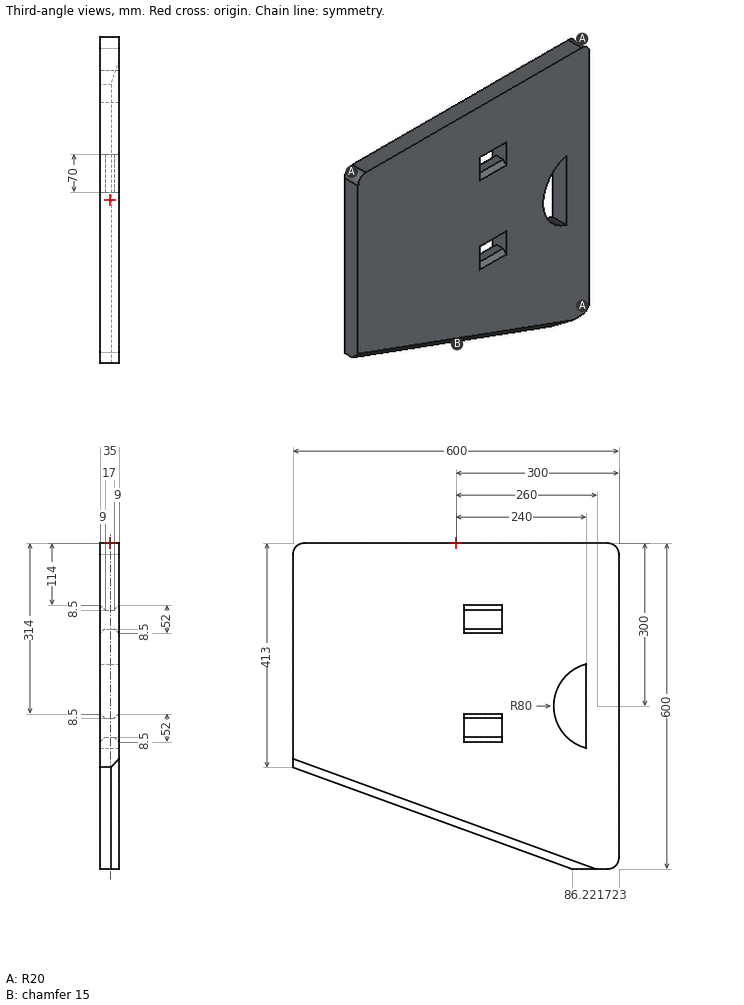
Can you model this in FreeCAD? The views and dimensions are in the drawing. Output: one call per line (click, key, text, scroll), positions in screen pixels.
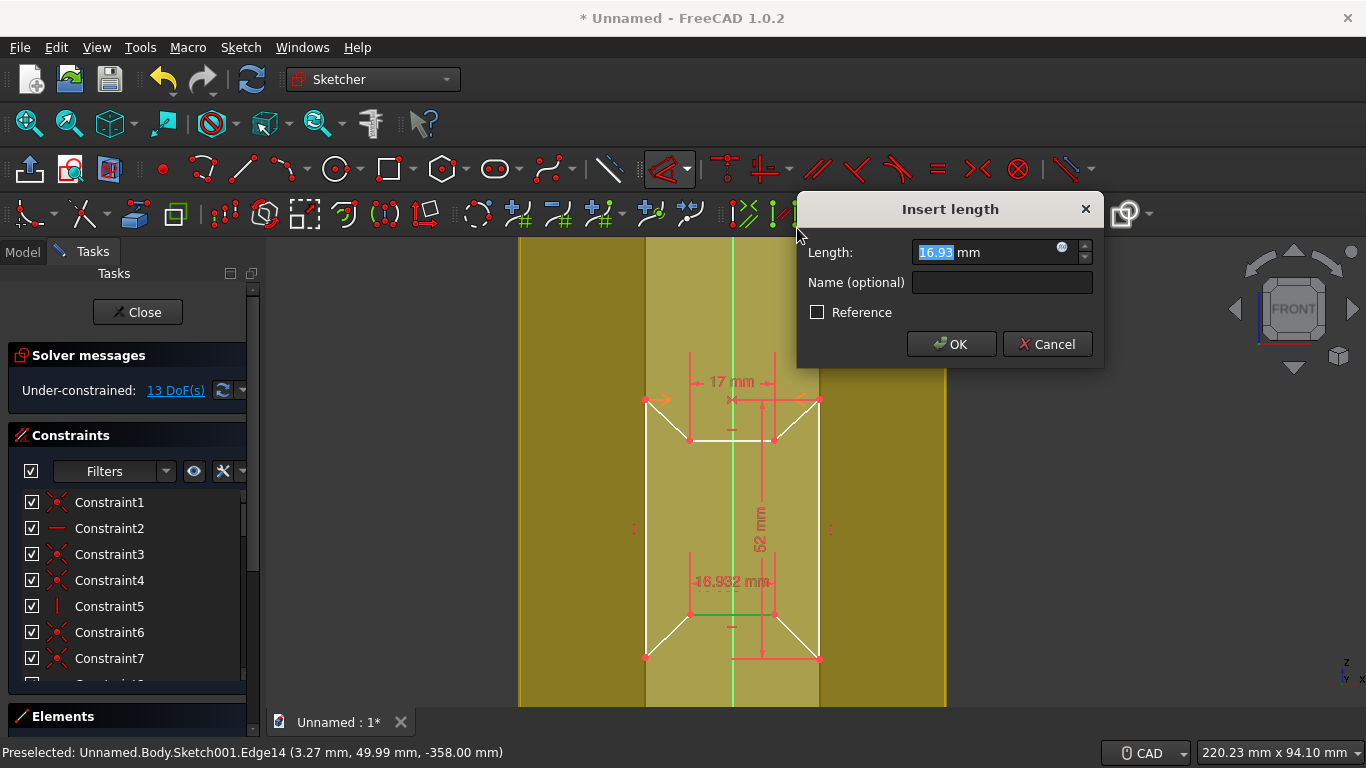
text(17)
key(Return)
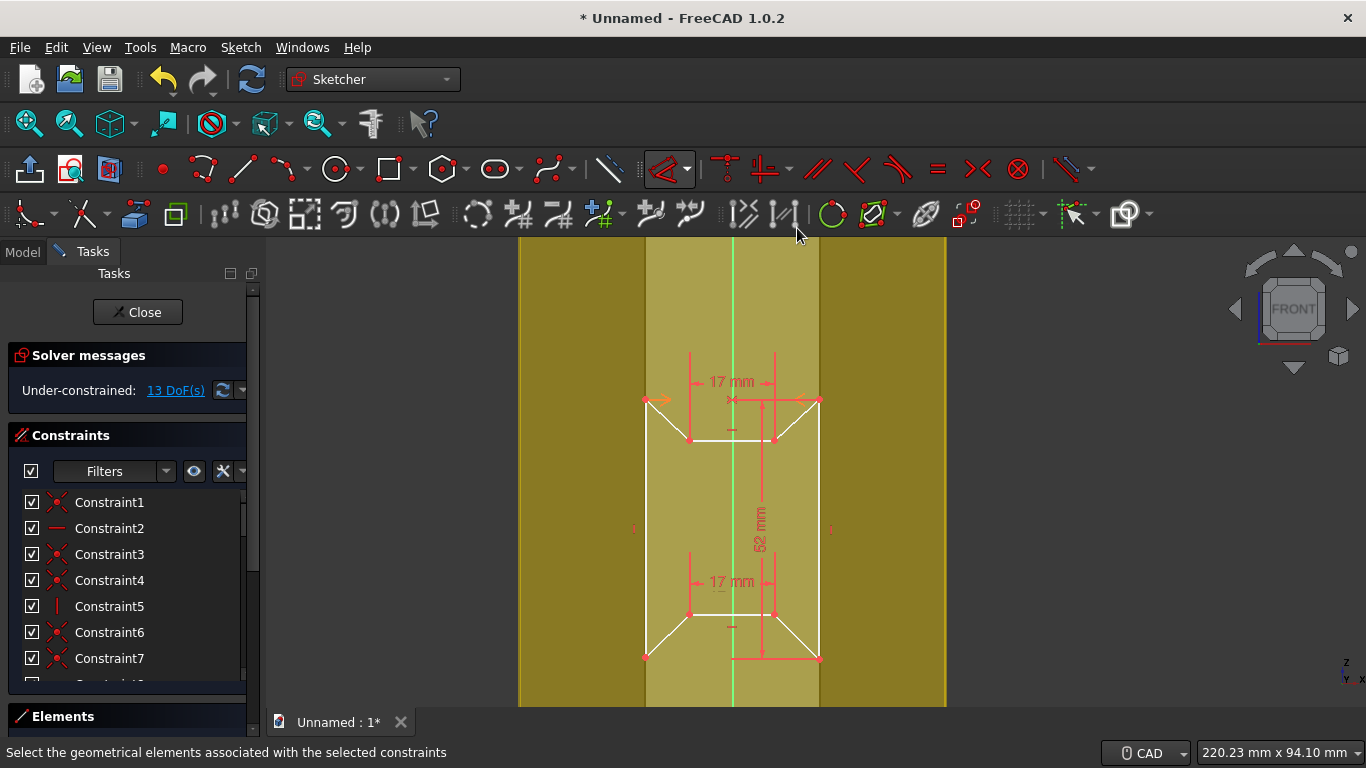
scroll(750, 617, down, 9)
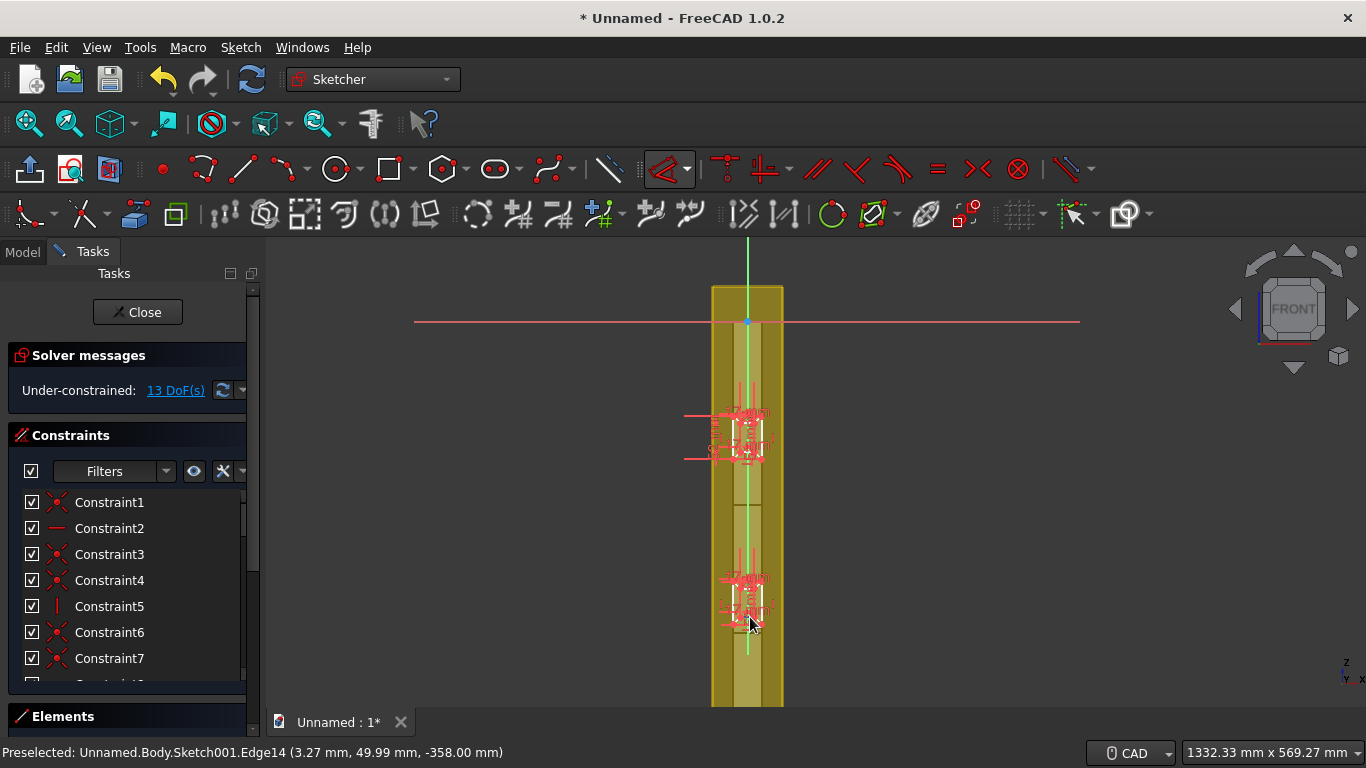
scroll(733, 612, up, 3)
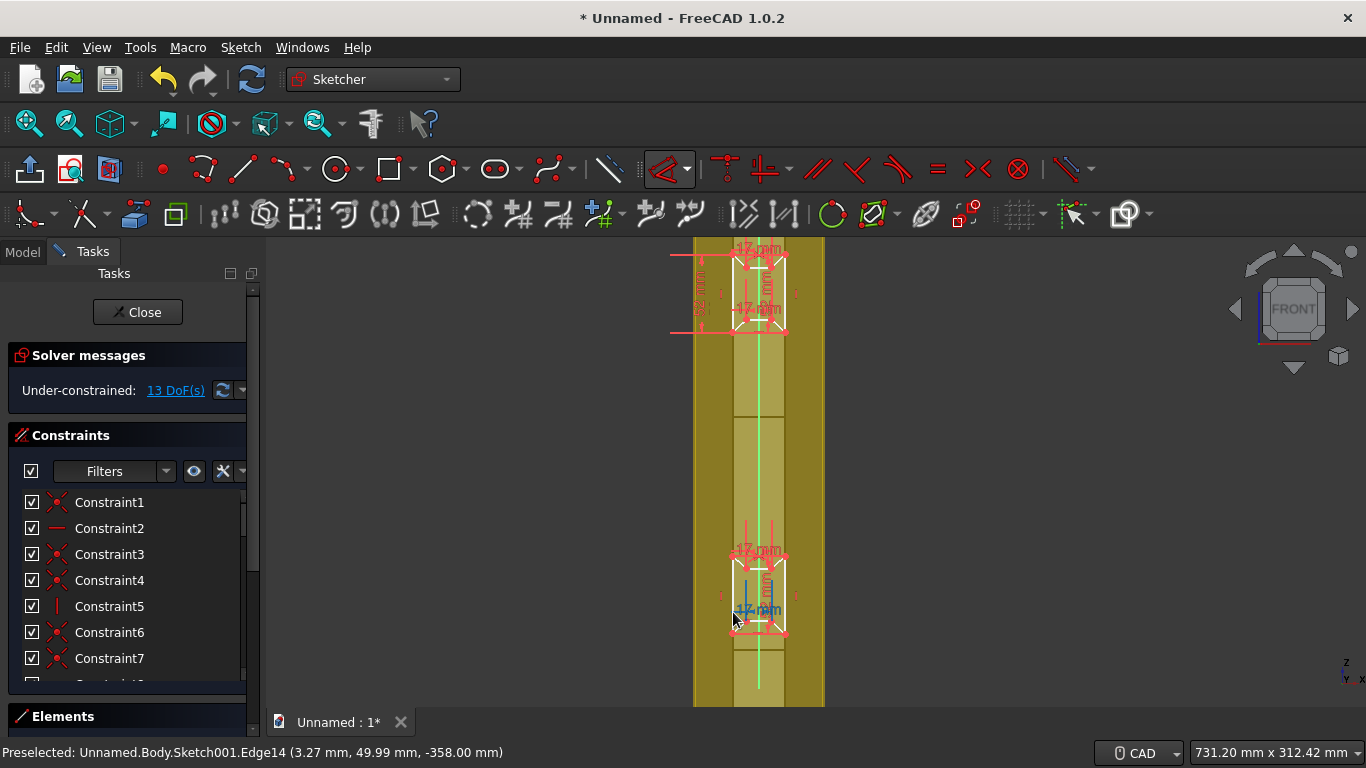
click(733, 611)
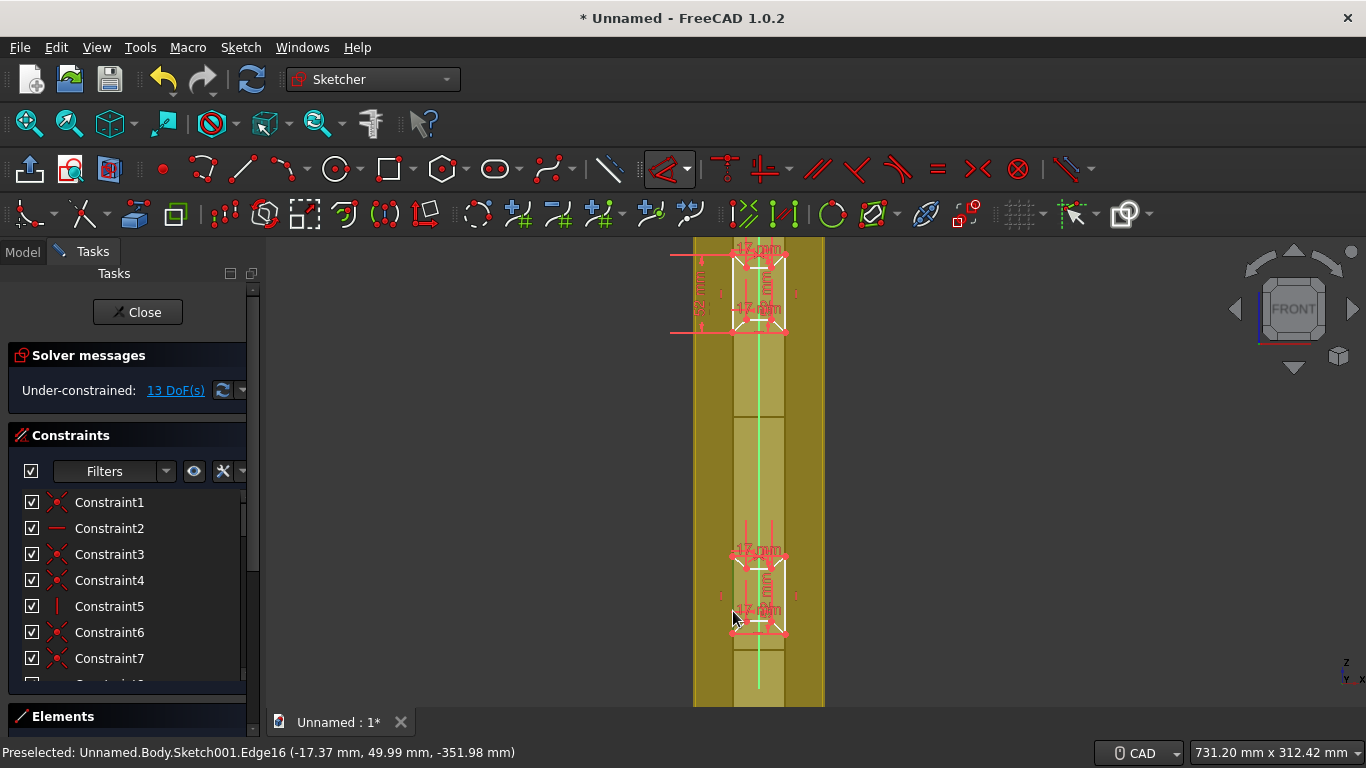
key(i)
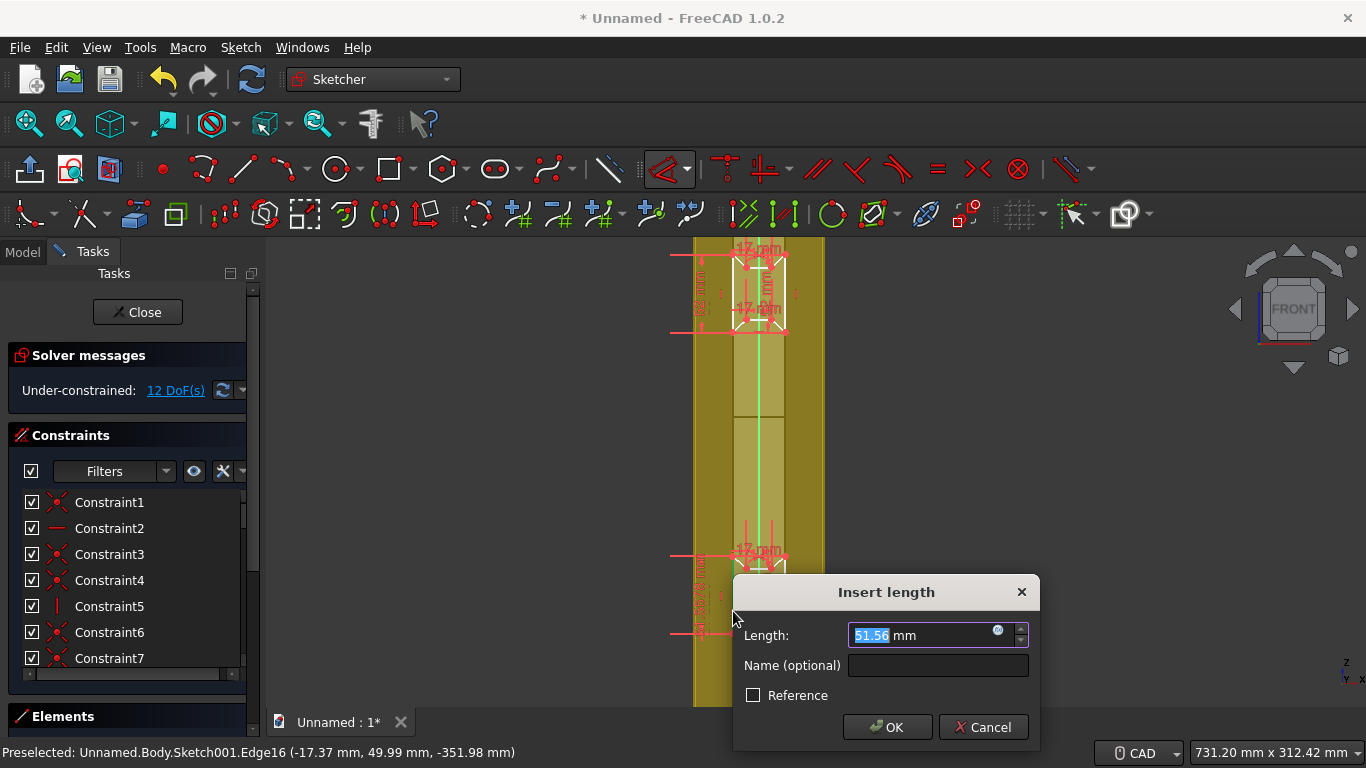
text(52)
key(Return)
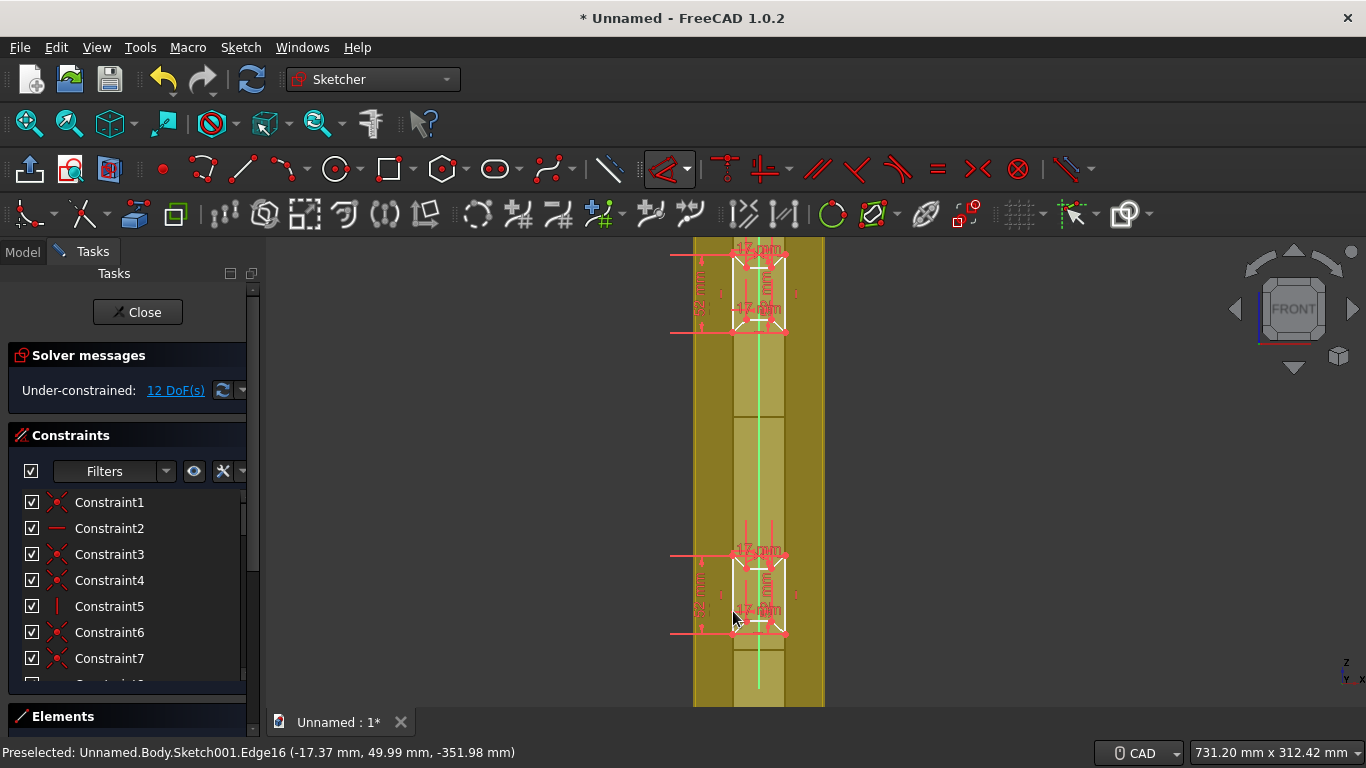
scroll(733, 611, down, 3)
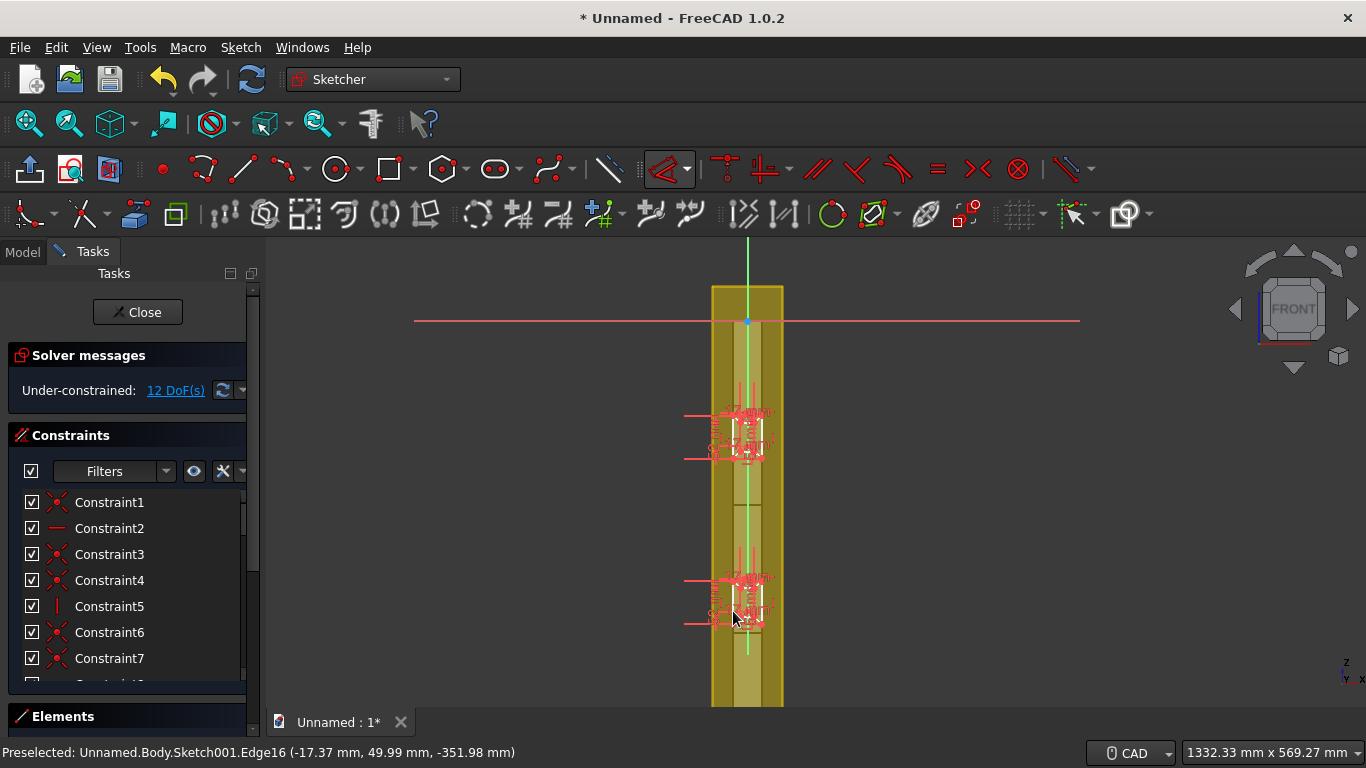
scroll(738, 420, up, 9)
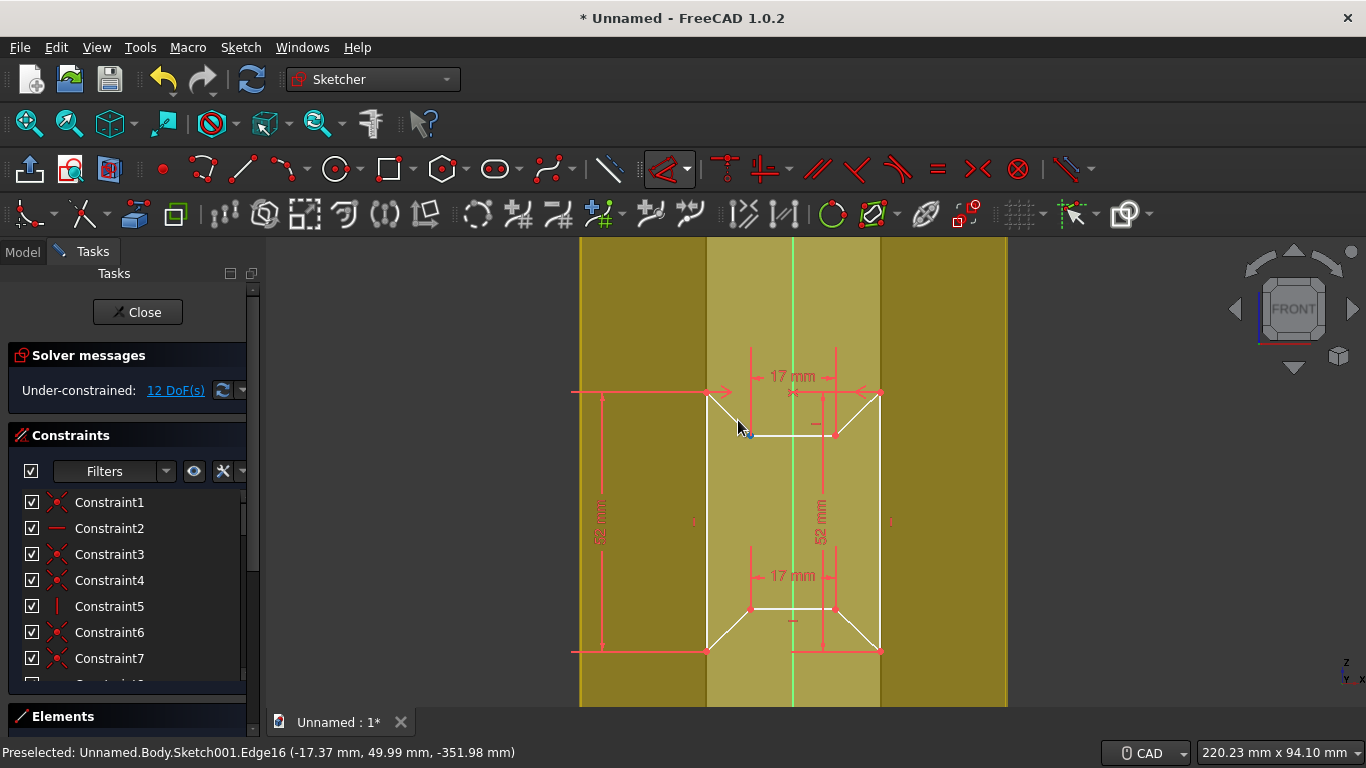
click(733, 418)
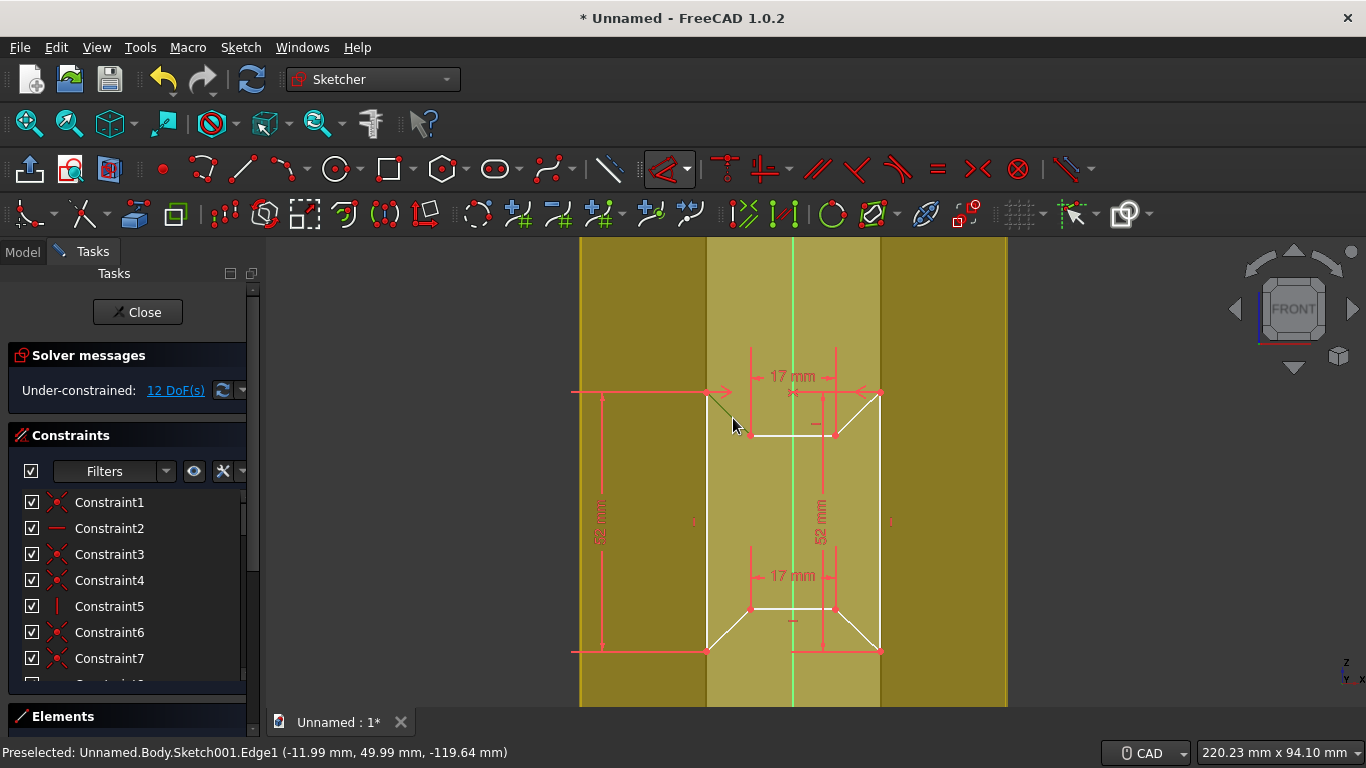
key(l)